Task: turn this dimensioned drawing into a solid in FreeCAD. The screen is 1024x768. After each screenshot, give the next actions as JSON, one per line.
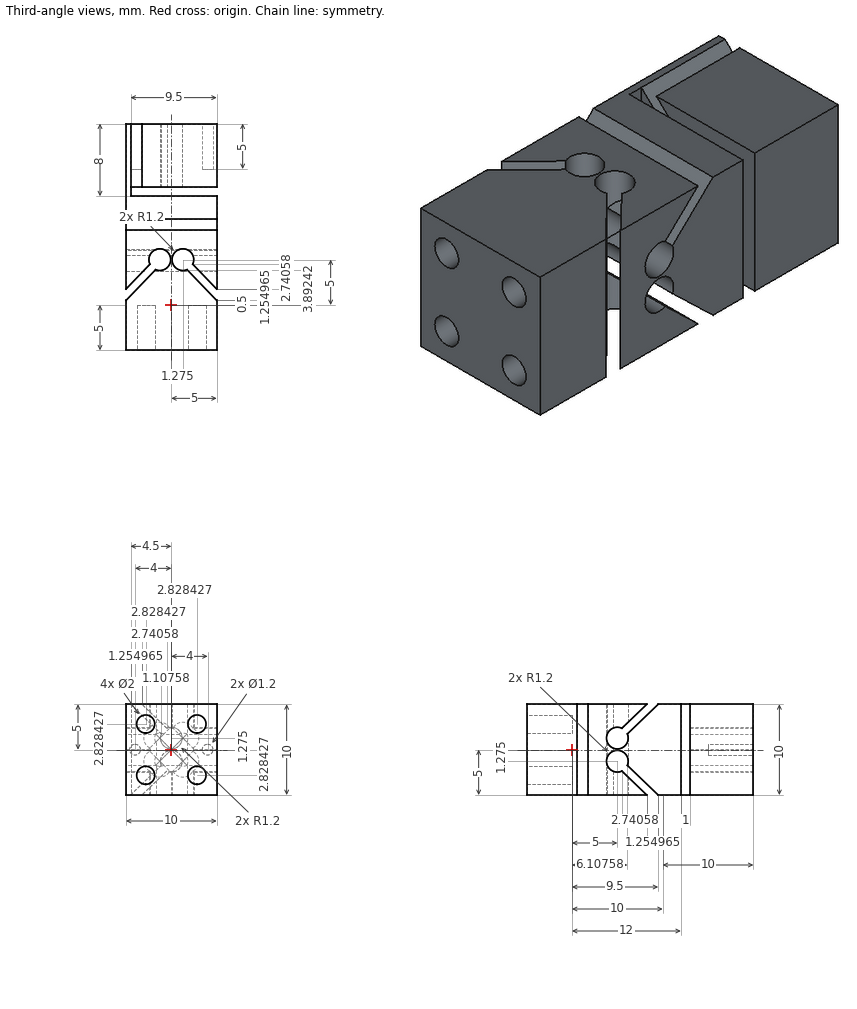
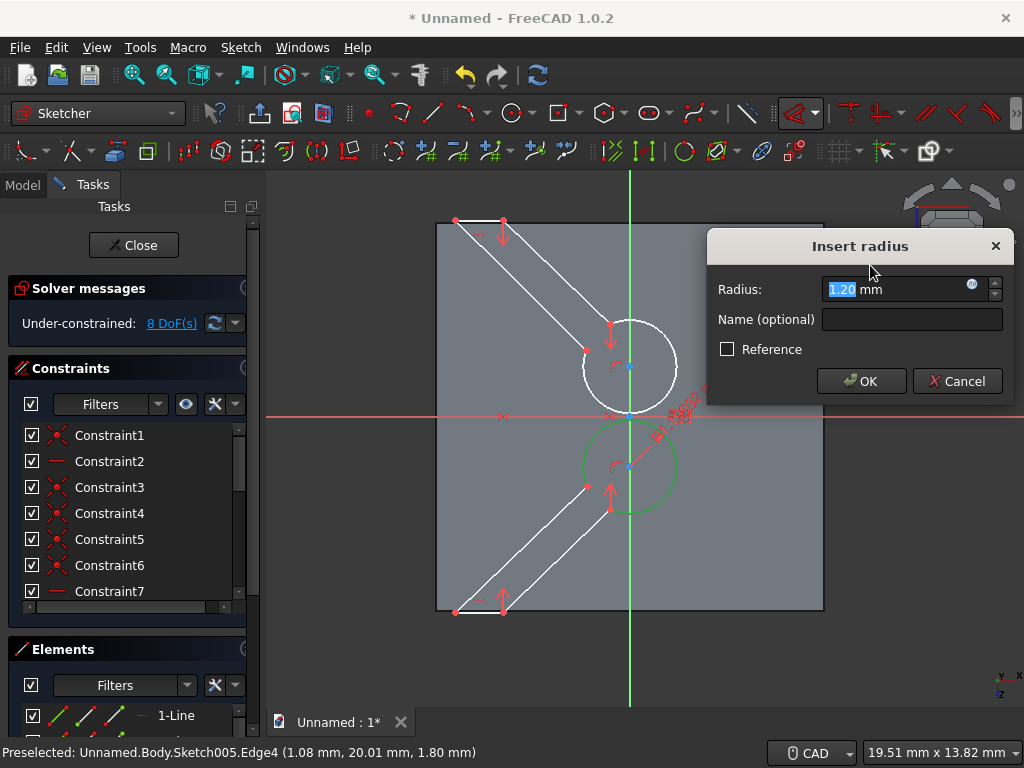
{"action": "type", "text": "1.2"}
{"action": "key", "text": "Return"}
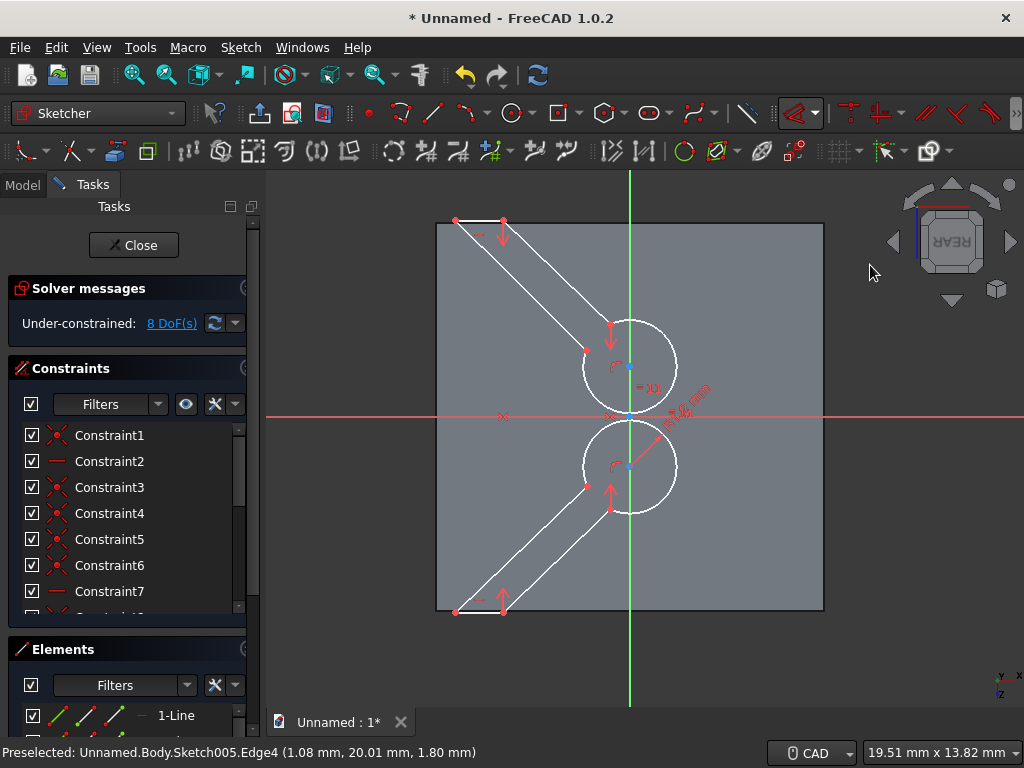
{"action": "left_click", "coordinate": [455, 613]}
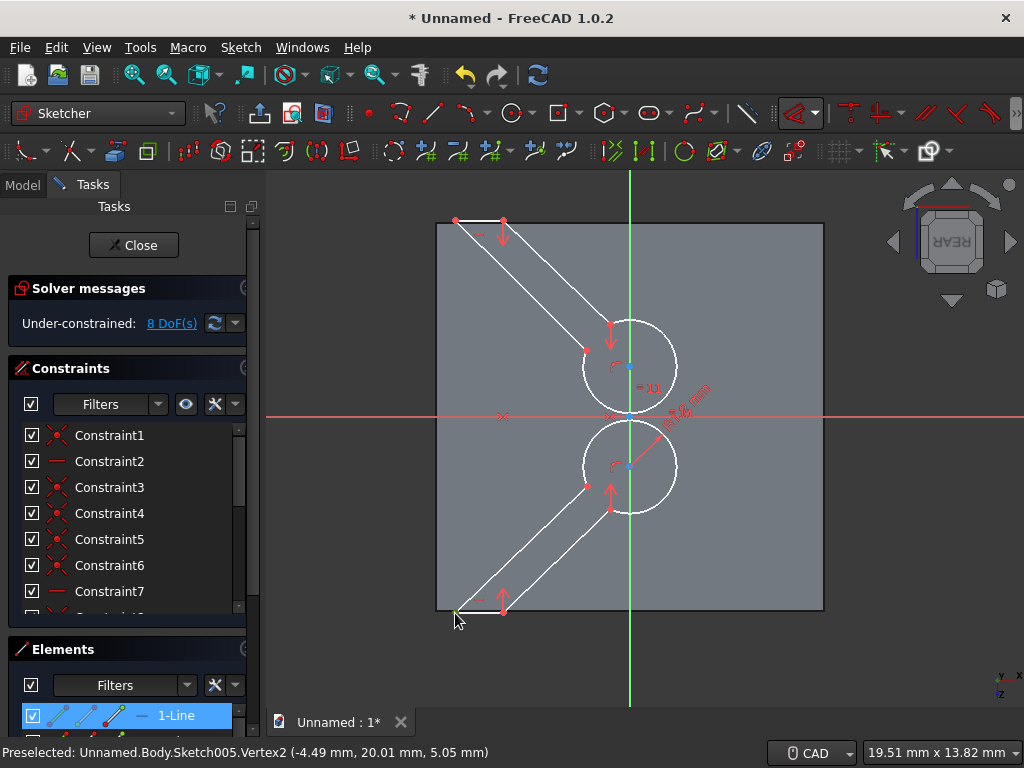
{"action": "left_click", "coordinate": [818, 114]}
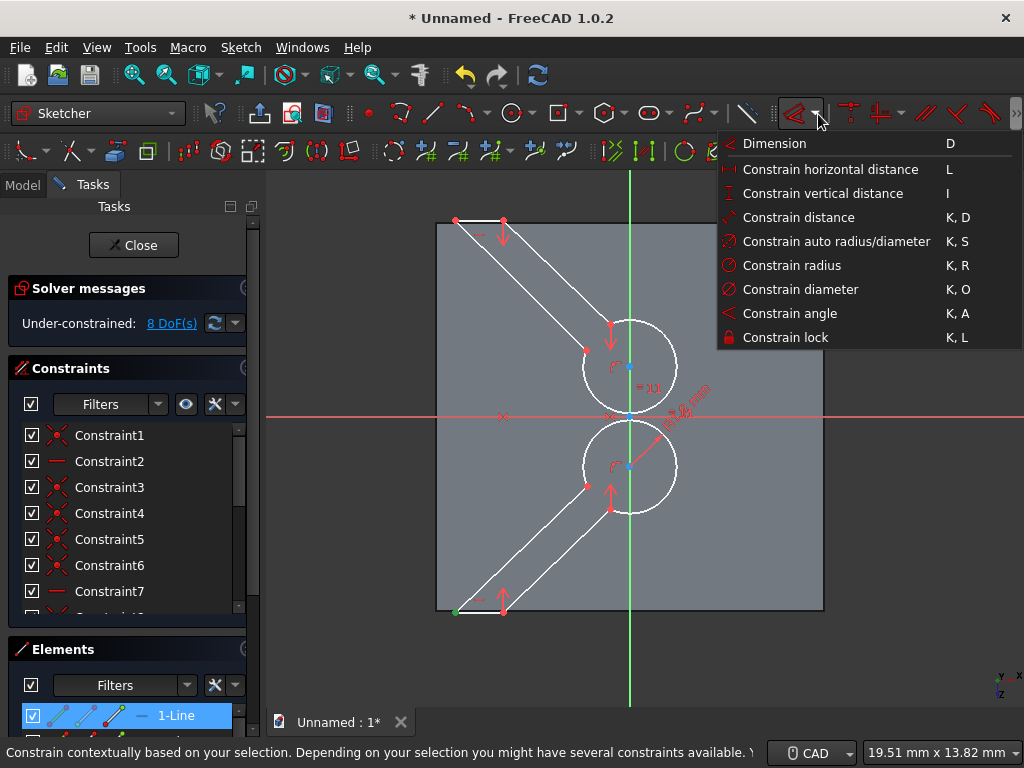
{"action": "left_click", "coordinate": [870, 193]}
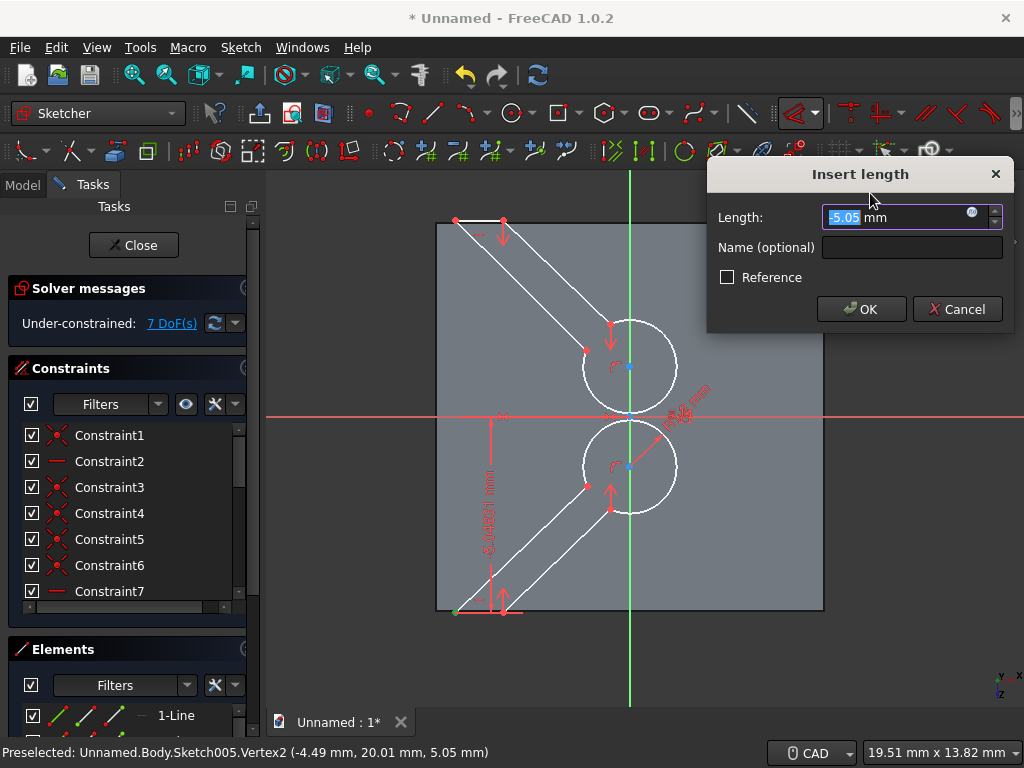
{"action": "type", "text": "-5"}
{"action": "key", "text": "Return"}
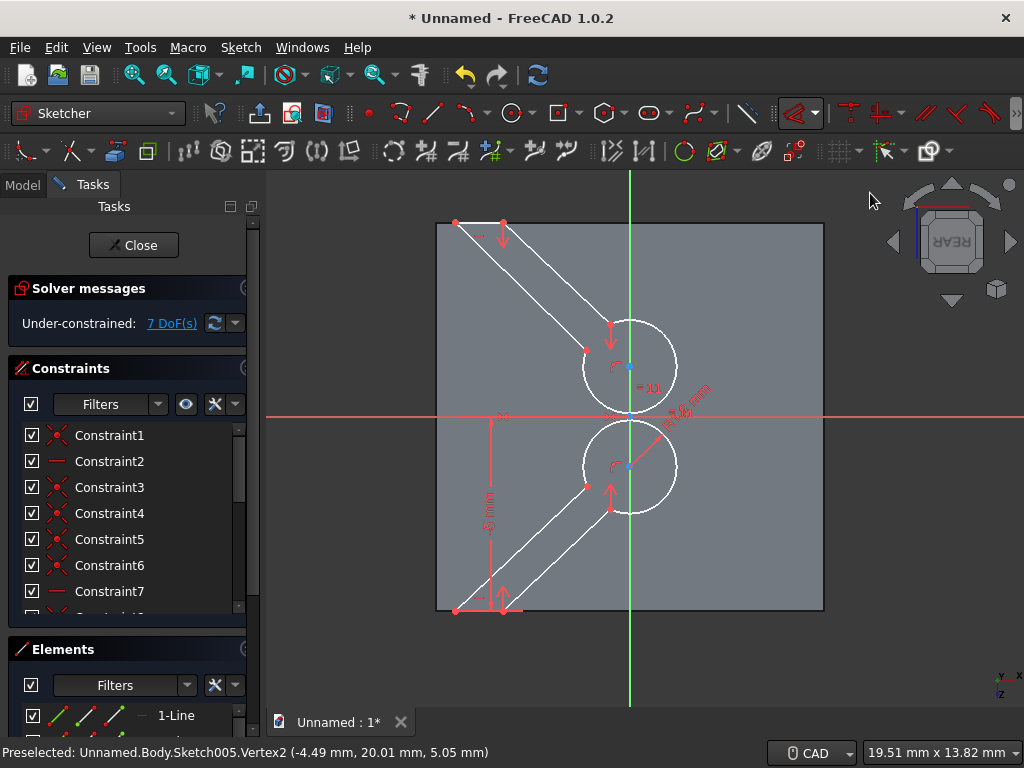
{"action": "left_click", "coordinate": [455, 611]}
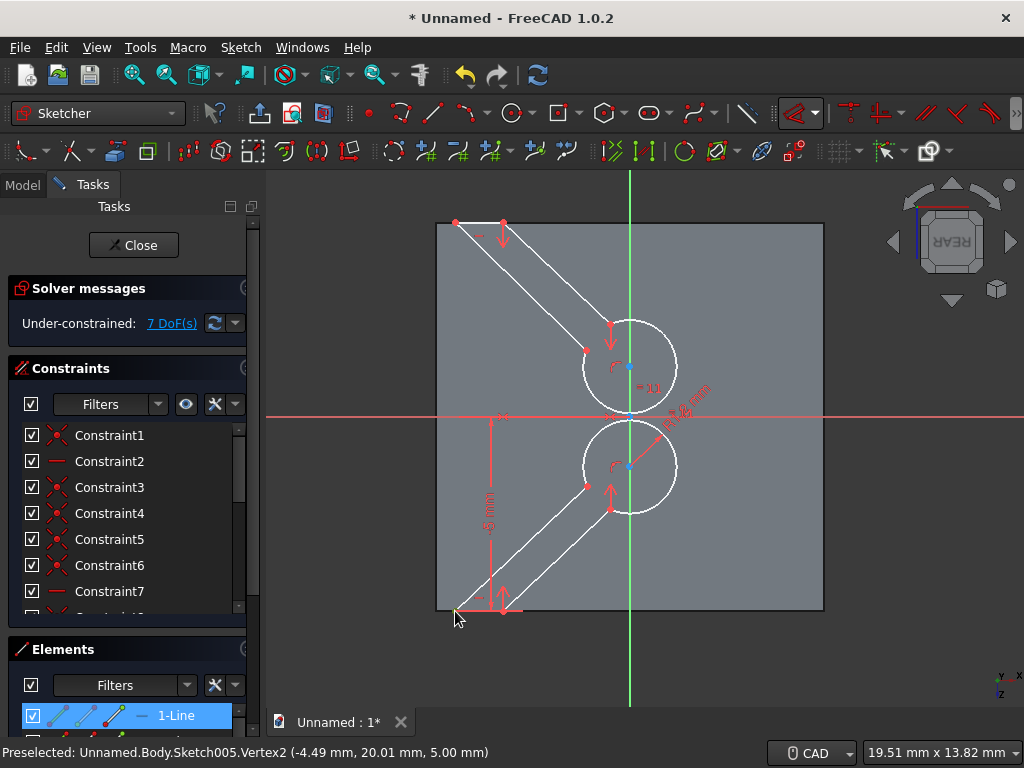
{"action": "left_click", "coordinate": [818, 114]}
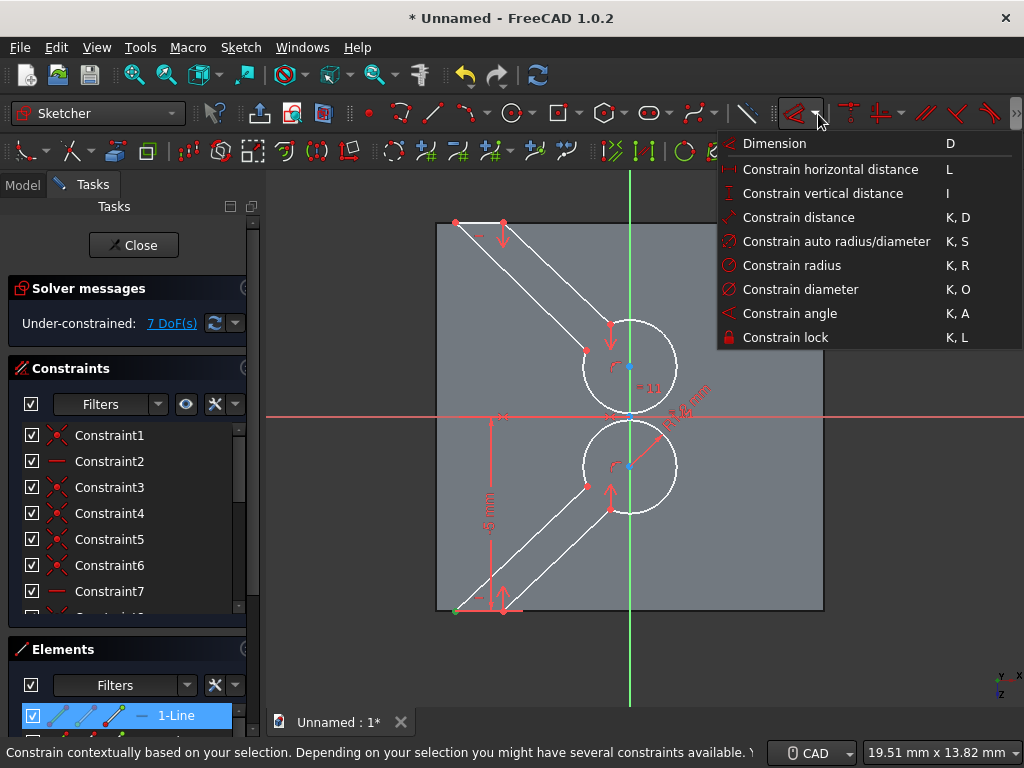
{"action": "left_click", "coordinate": [870, 169]}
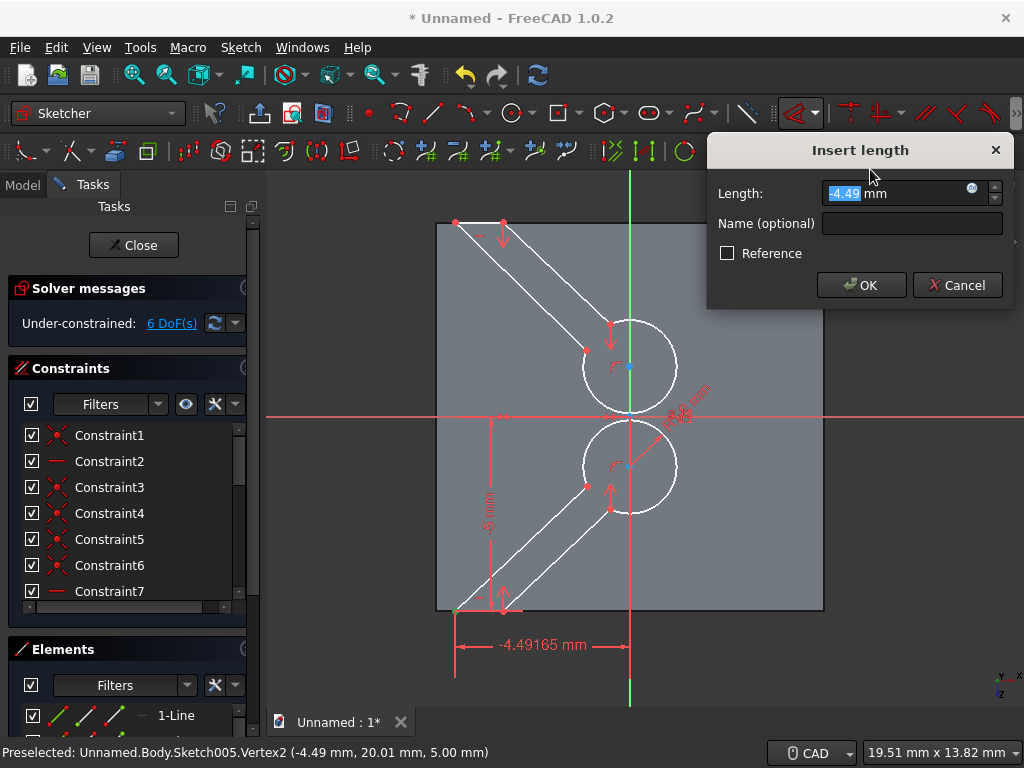
{"action": "type", "text": "-4.5"}
{"action": "key", "text": "Return"}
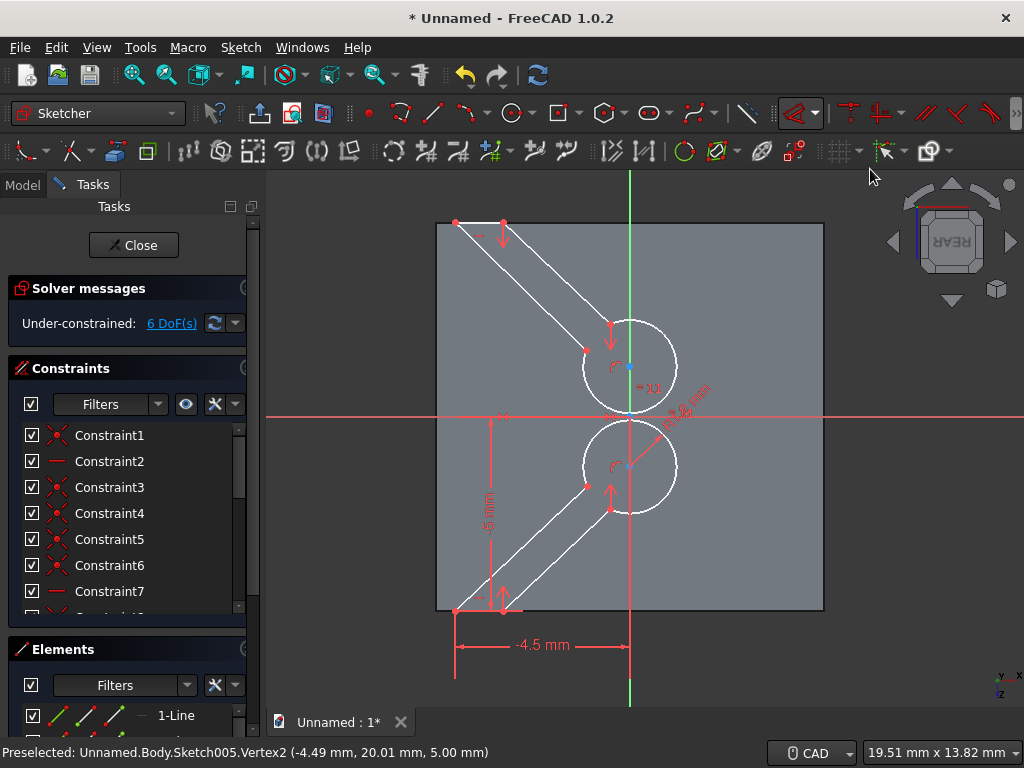
{"action": "left_click", "coordinate": [455, 223]}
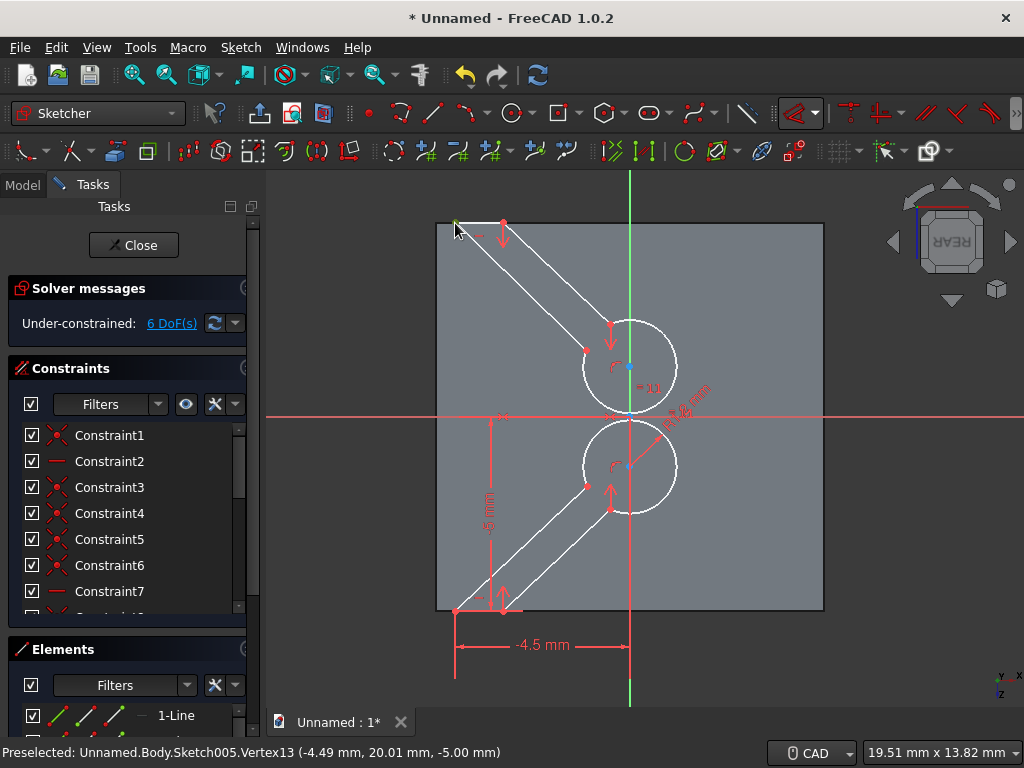
{"action": "left_click", "coordinate": [818, 114]}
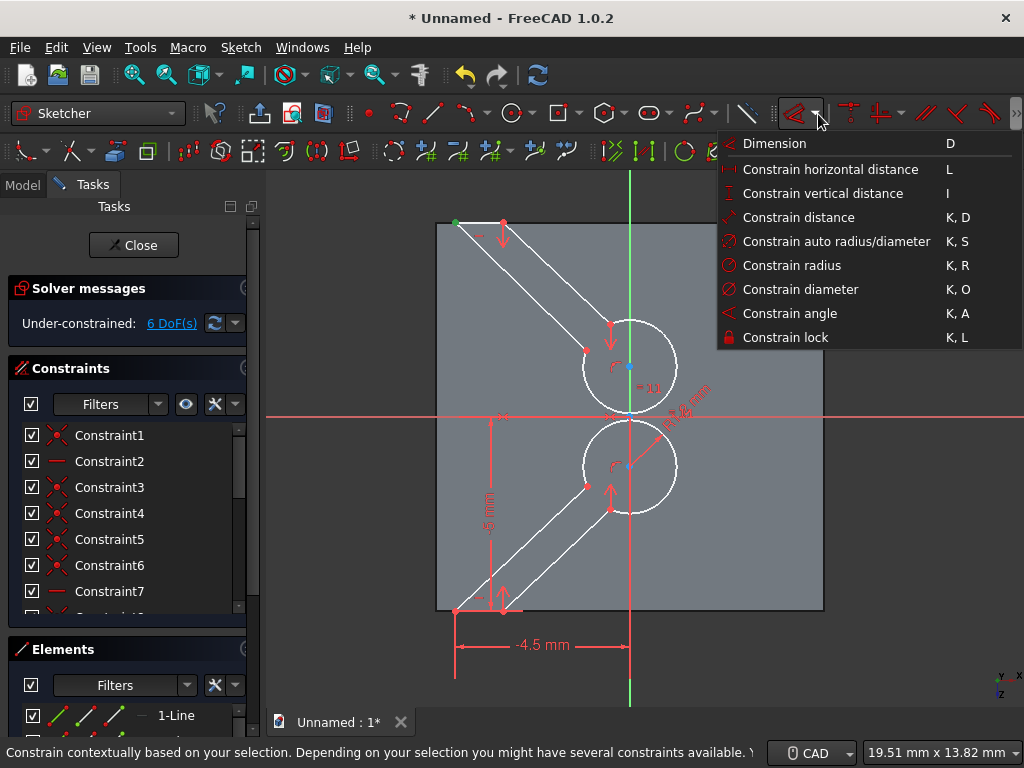
{"action": "left_click", "coordinate": [870, 169]}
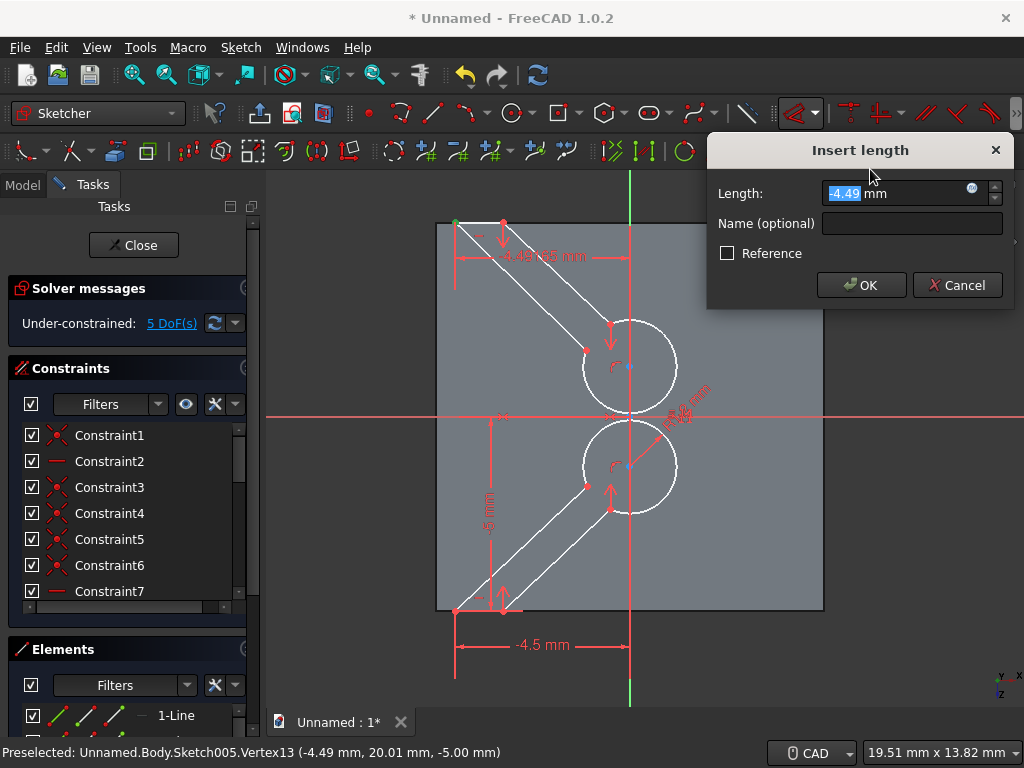
{"action": "type", "text": "-4.5"}
{"action": "key", "text": "Return"}